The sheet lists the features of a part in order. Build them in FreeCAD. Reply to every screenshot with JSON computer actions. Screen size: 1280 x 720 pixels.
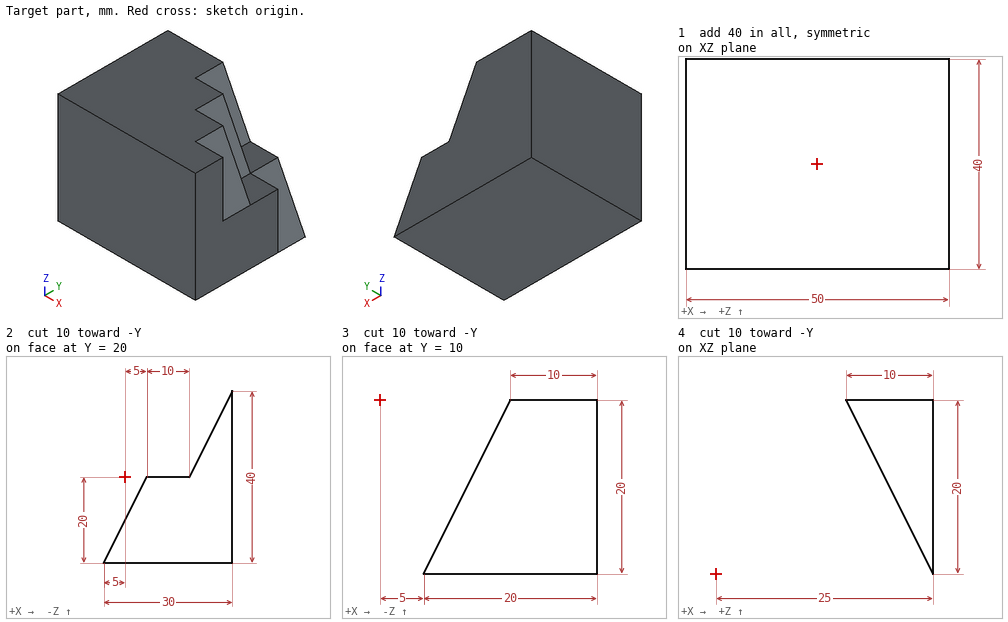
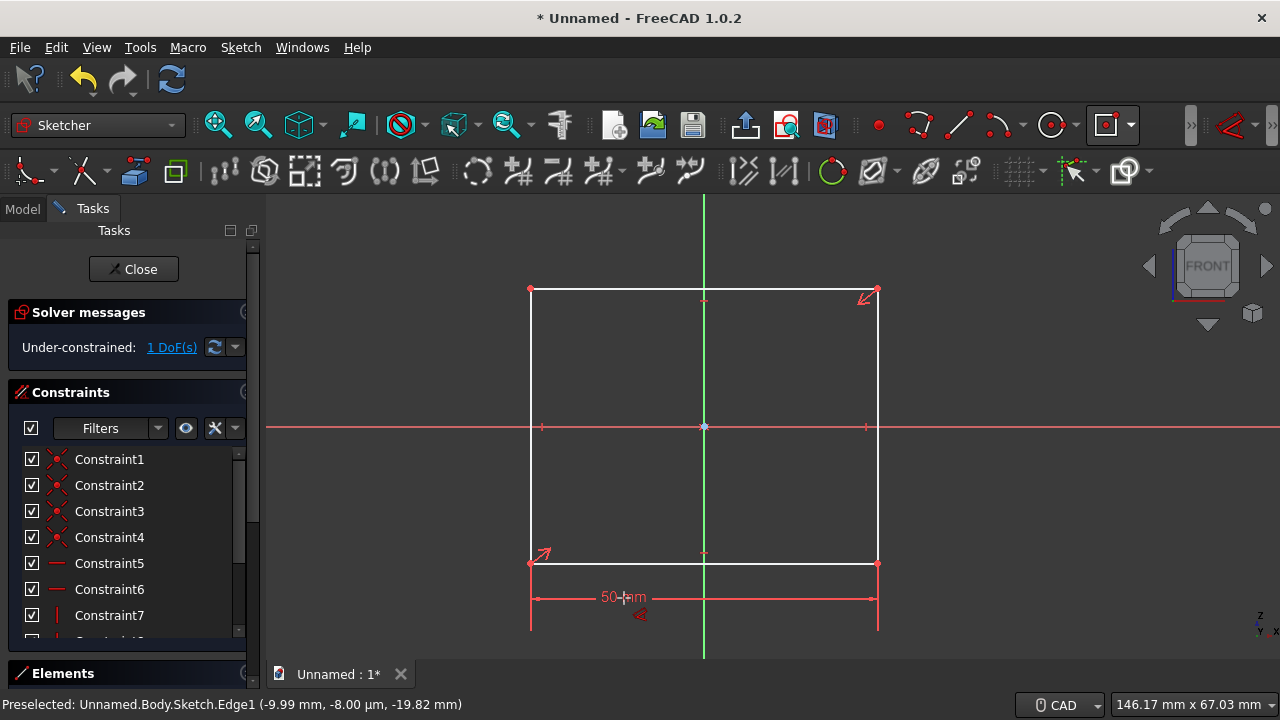
{"action": "left_click", "coordinate": [878, 482]}
{"action": "left_click", "coordinate": [912, 363]}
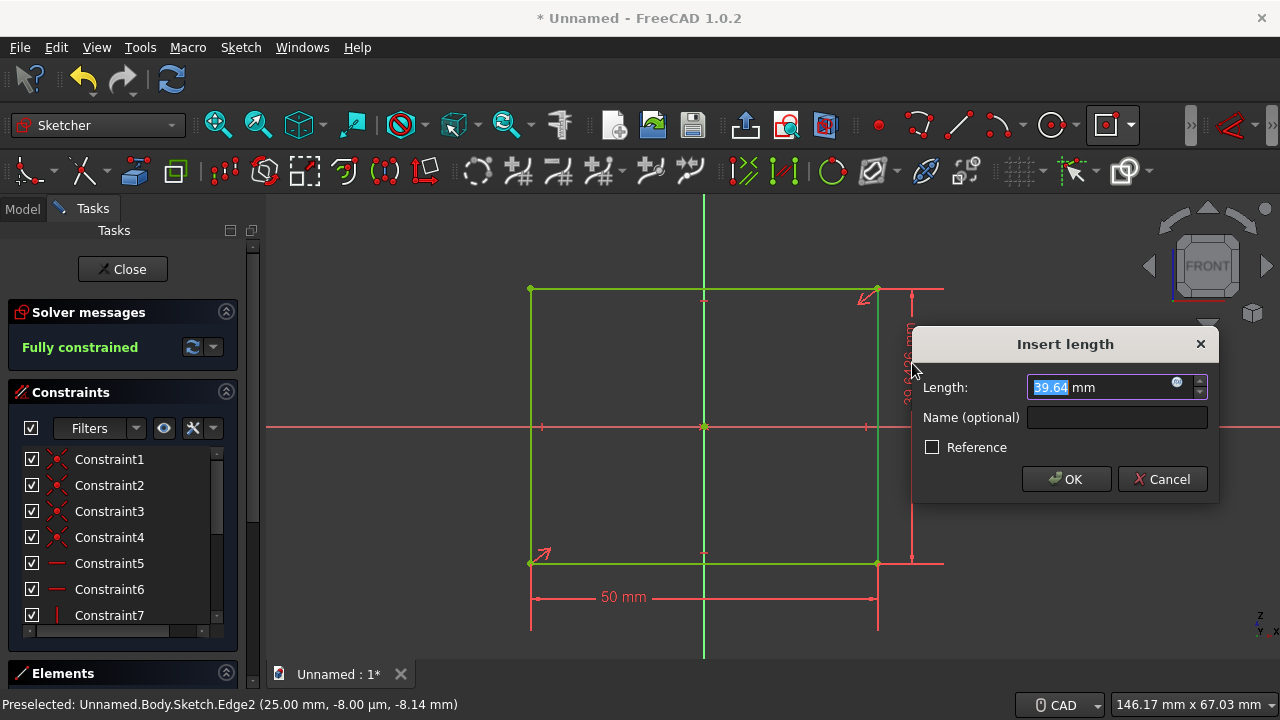
{"action": "type", "text": "40"}
{"action": "key", "text": "Return"}
{"action": "key", "text": "Escape"}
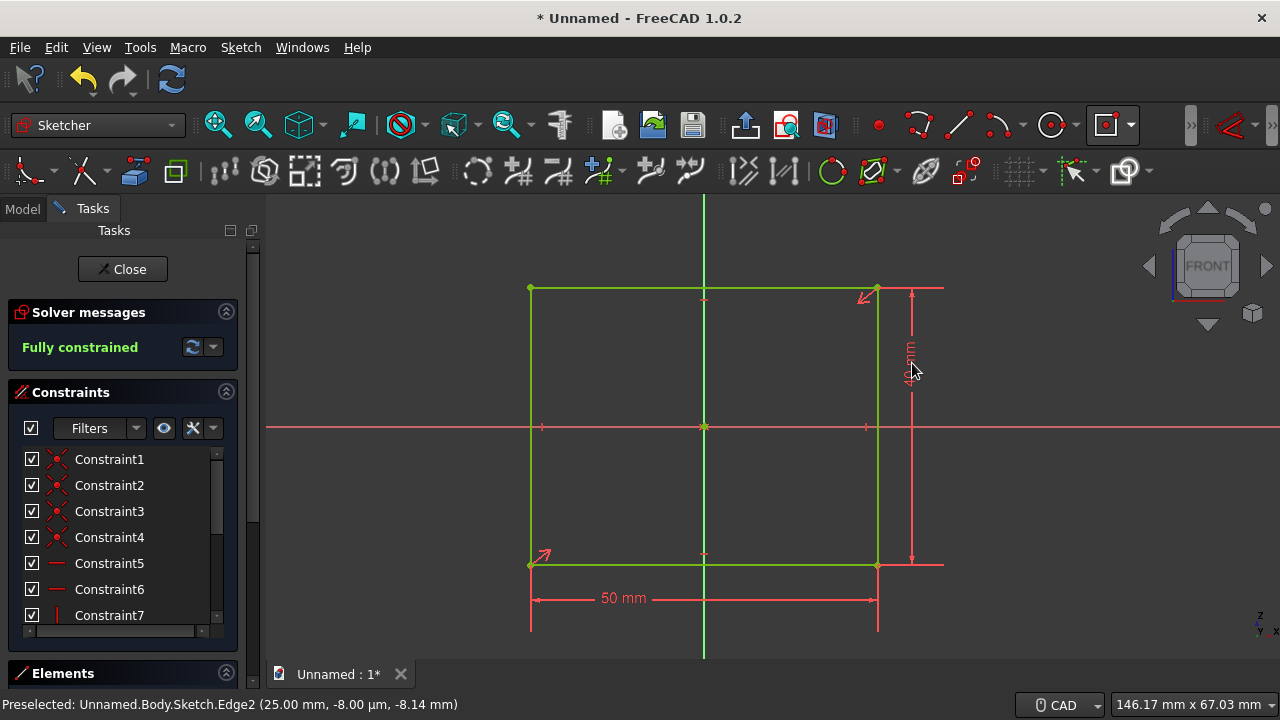
{"action": "left_click", "coordinate": [123, 269]}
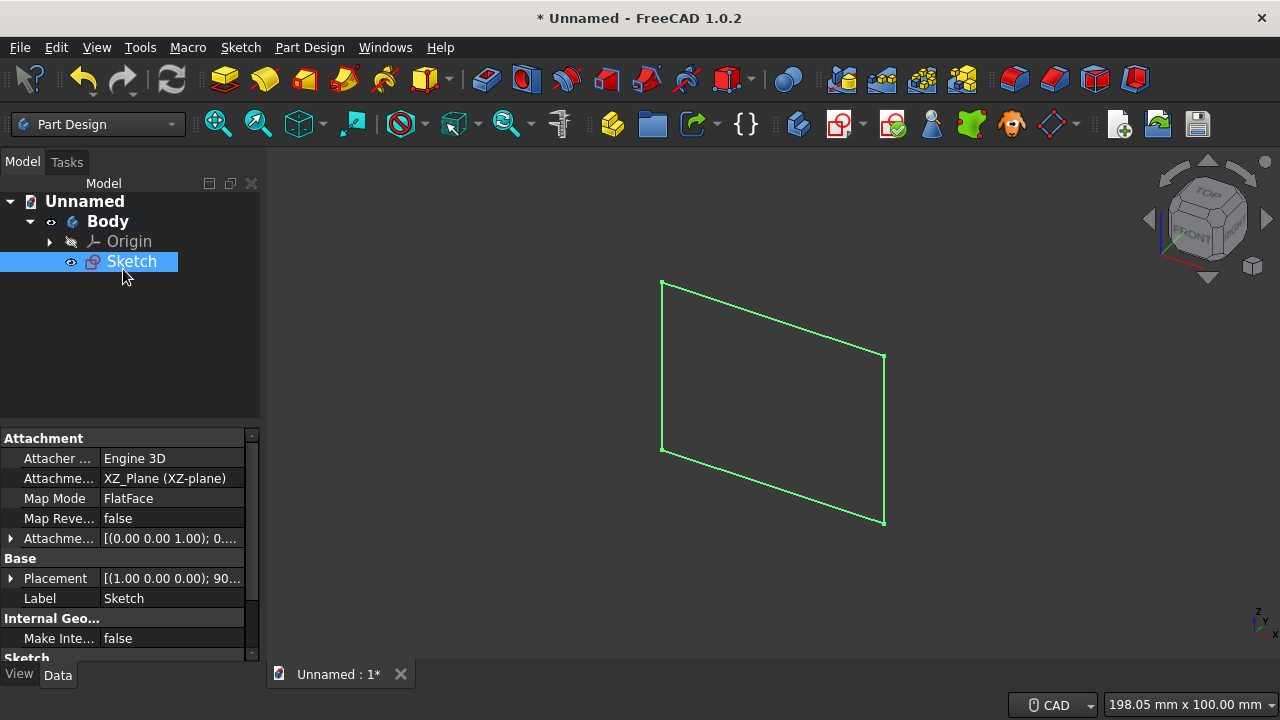
{"action": "left_click", "coordinate": [226, 80]}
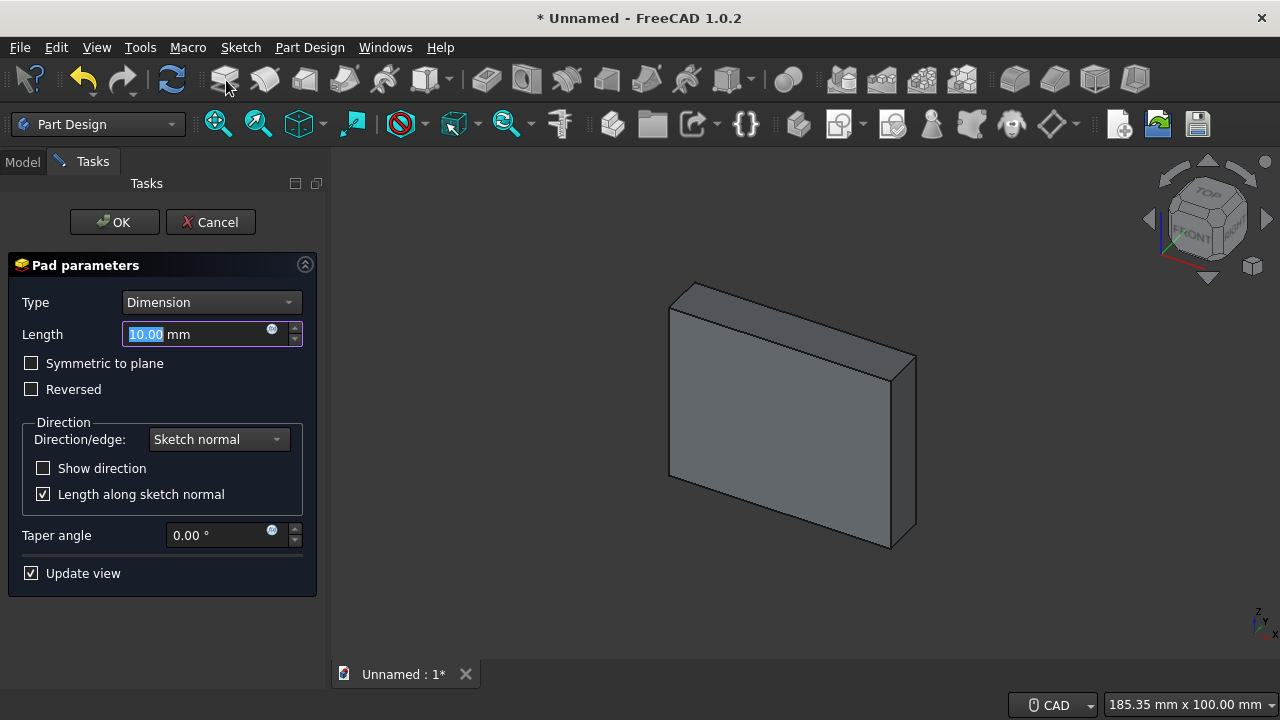
{"action": "type", "text": "40"}
{"action": "key", "text": "Tab"}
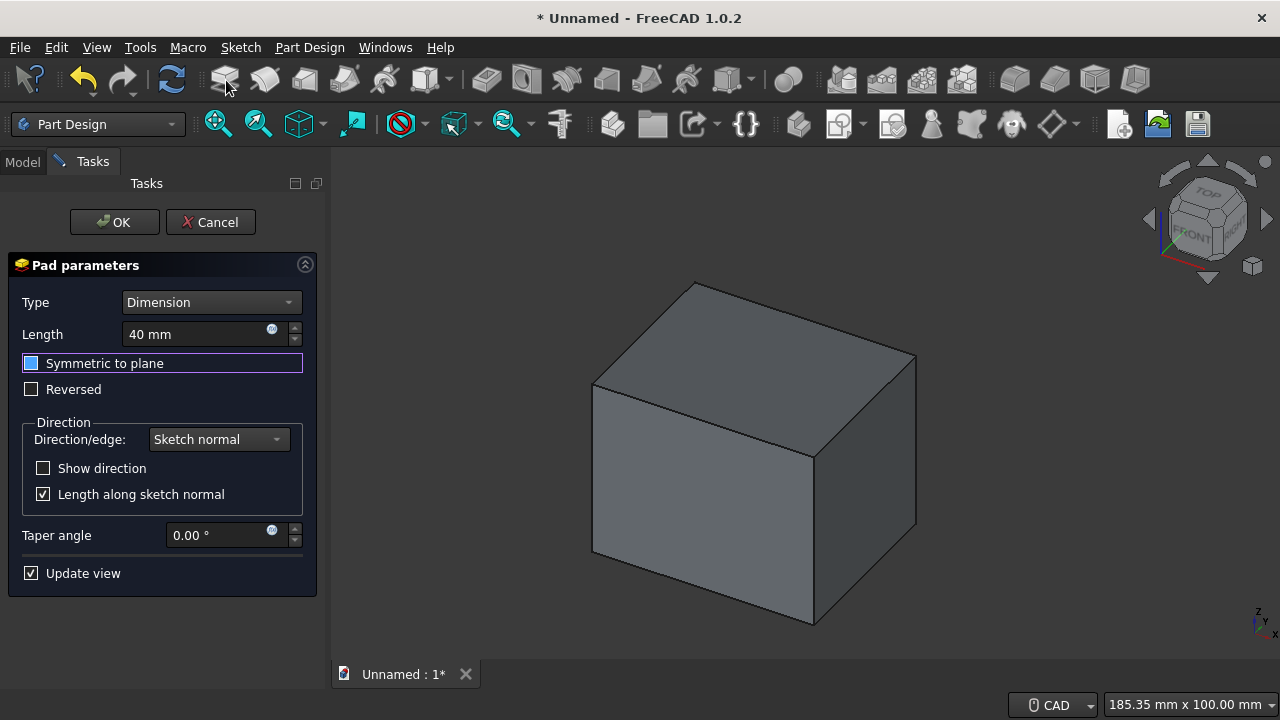
{"action": "left_click", "coordinate": [30, 363]}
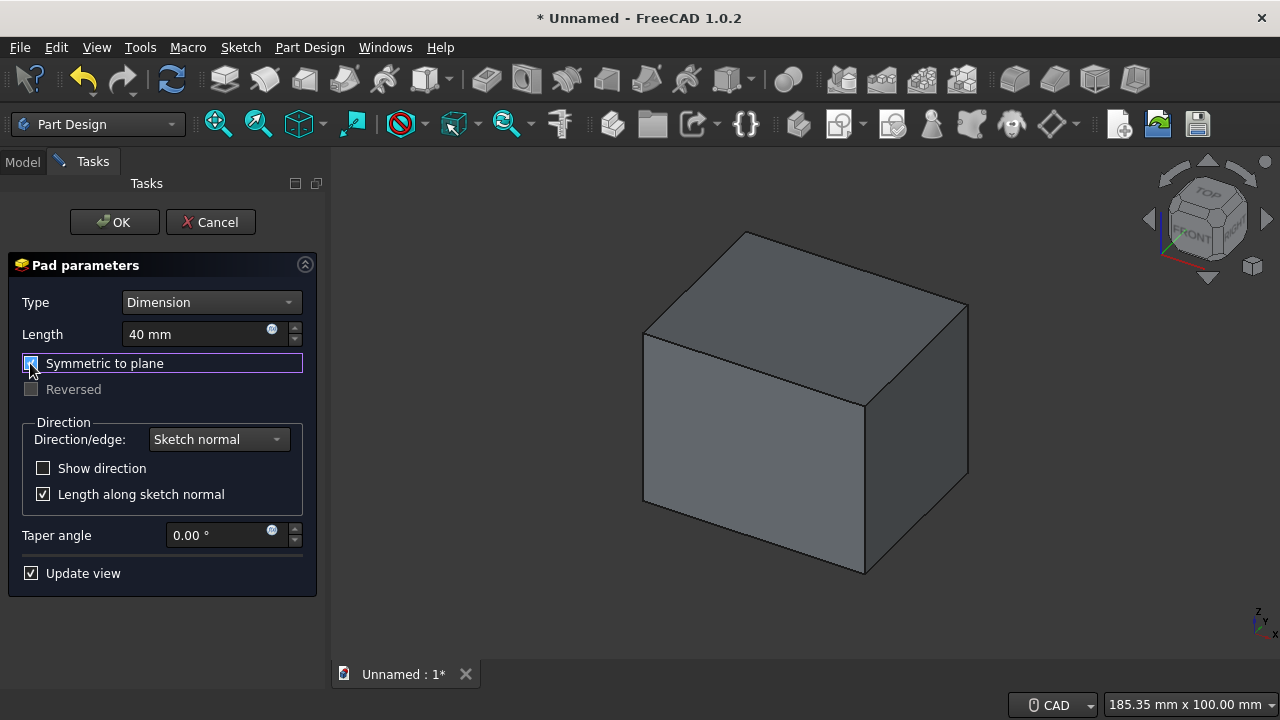
{"action": "left_click", "coordinate": [115, 222]}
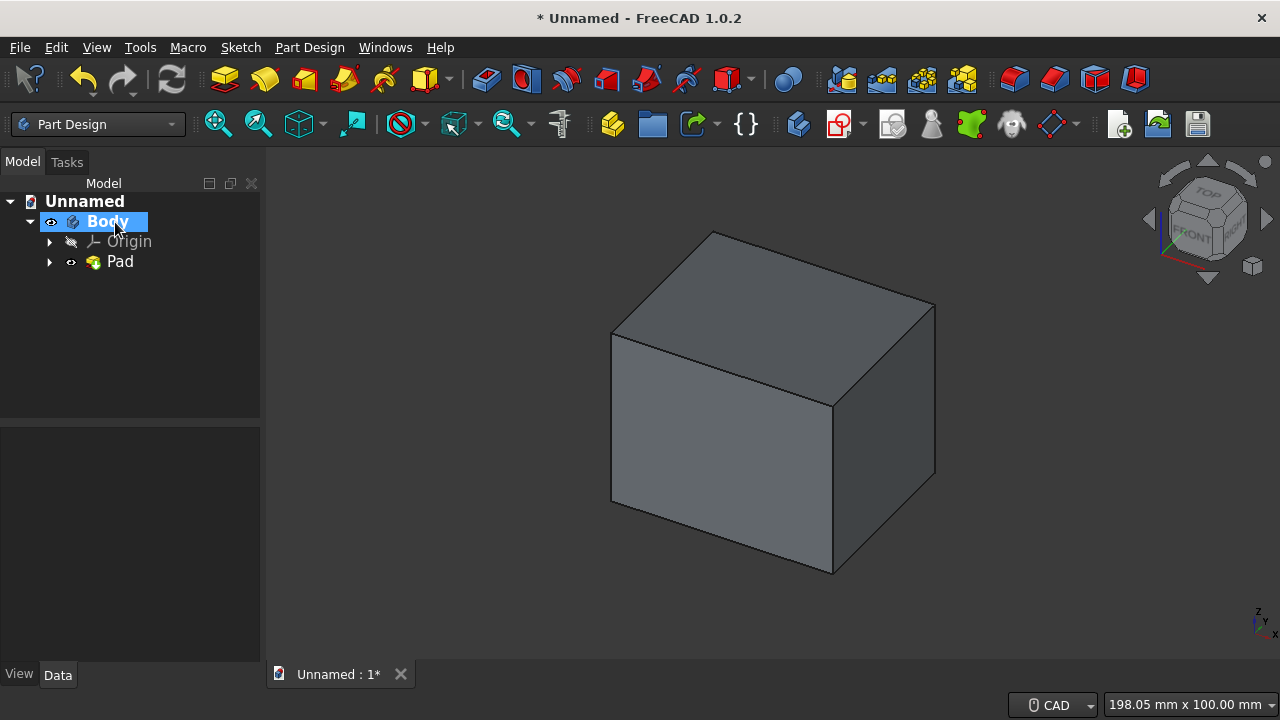
{"action": "key", "text": "4"}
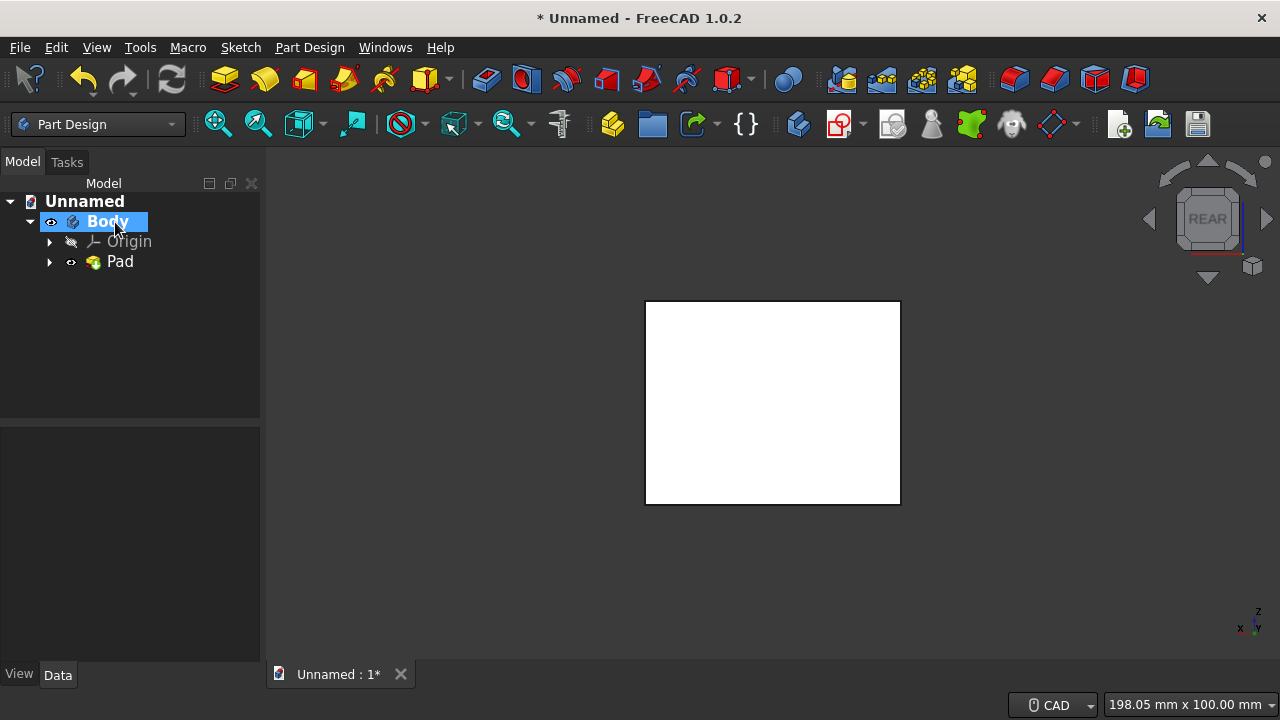
{"action": "left_click", "coordinate": [220, 124]}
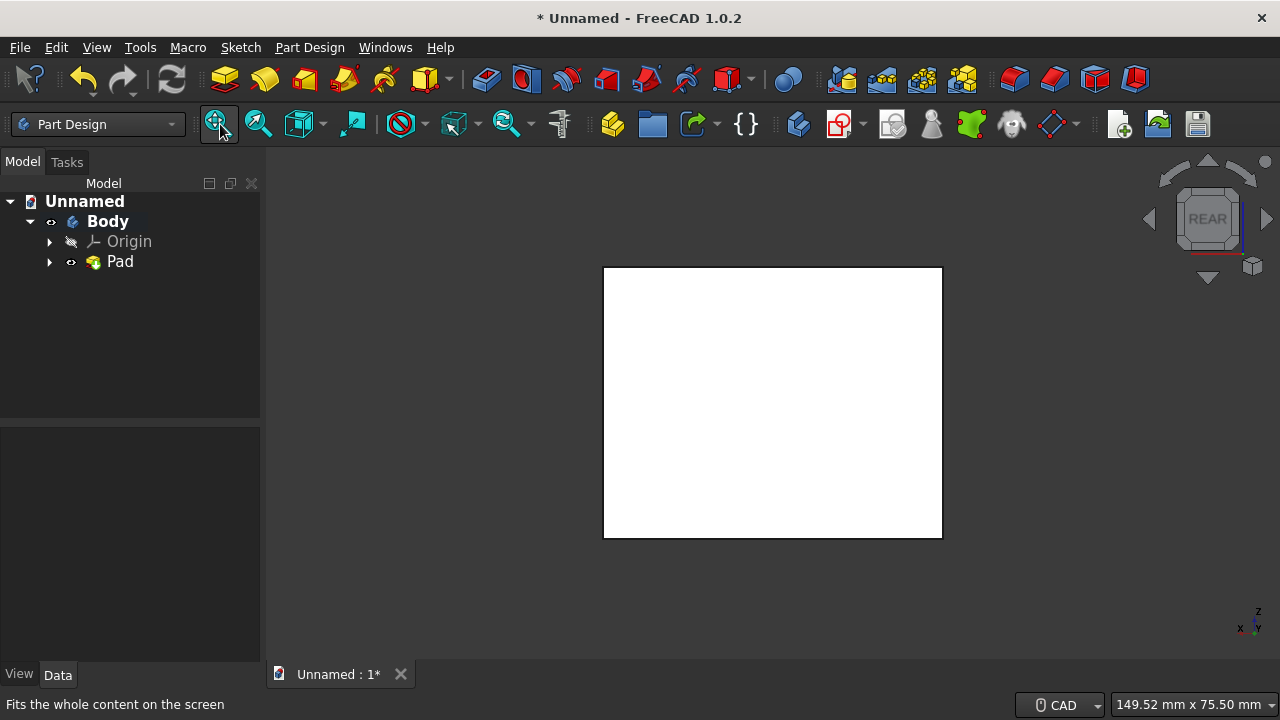
{"action": "left_click", "coordinate": [773, 402]}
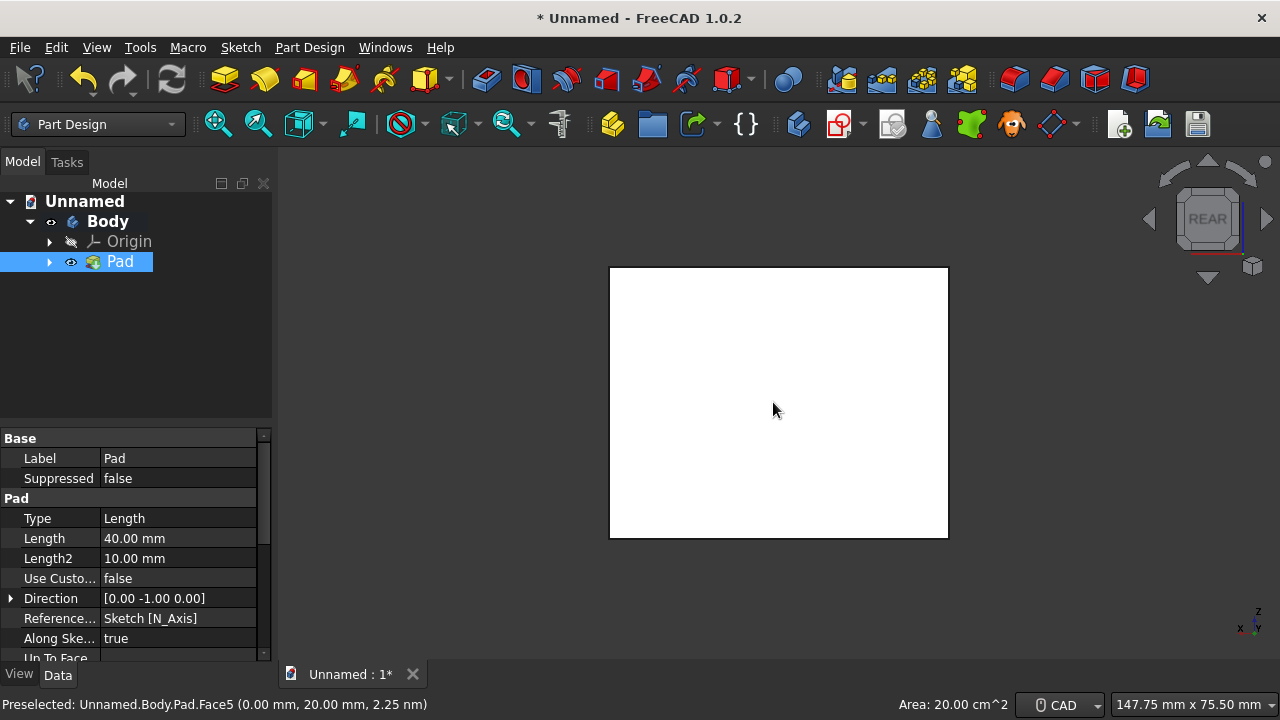
{"action": "left_click", "coordinate": [840, 124]}